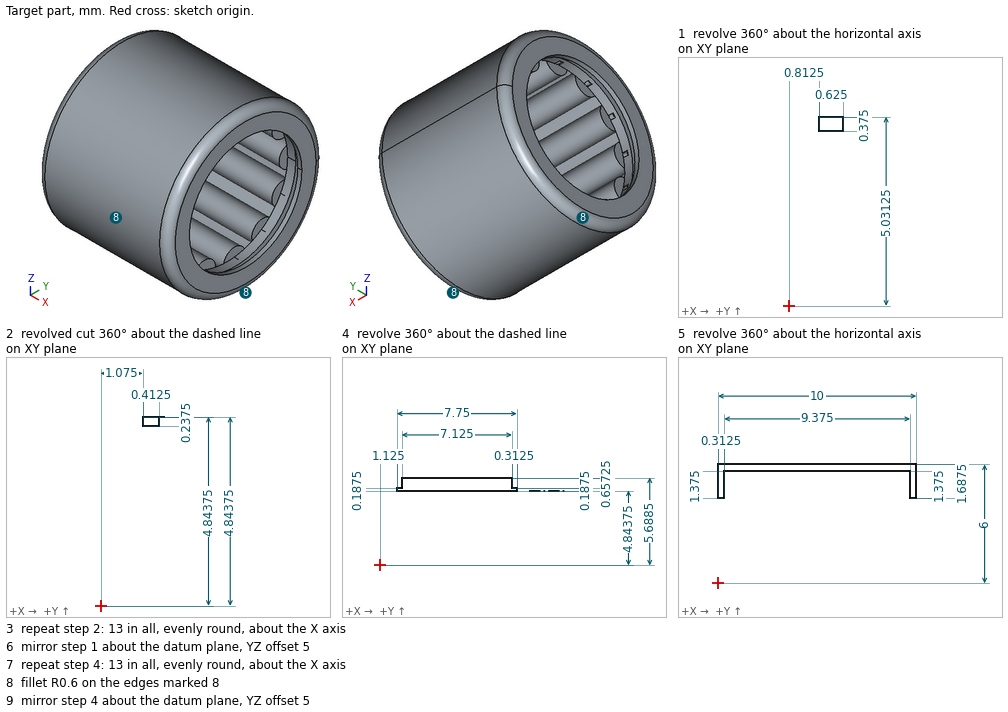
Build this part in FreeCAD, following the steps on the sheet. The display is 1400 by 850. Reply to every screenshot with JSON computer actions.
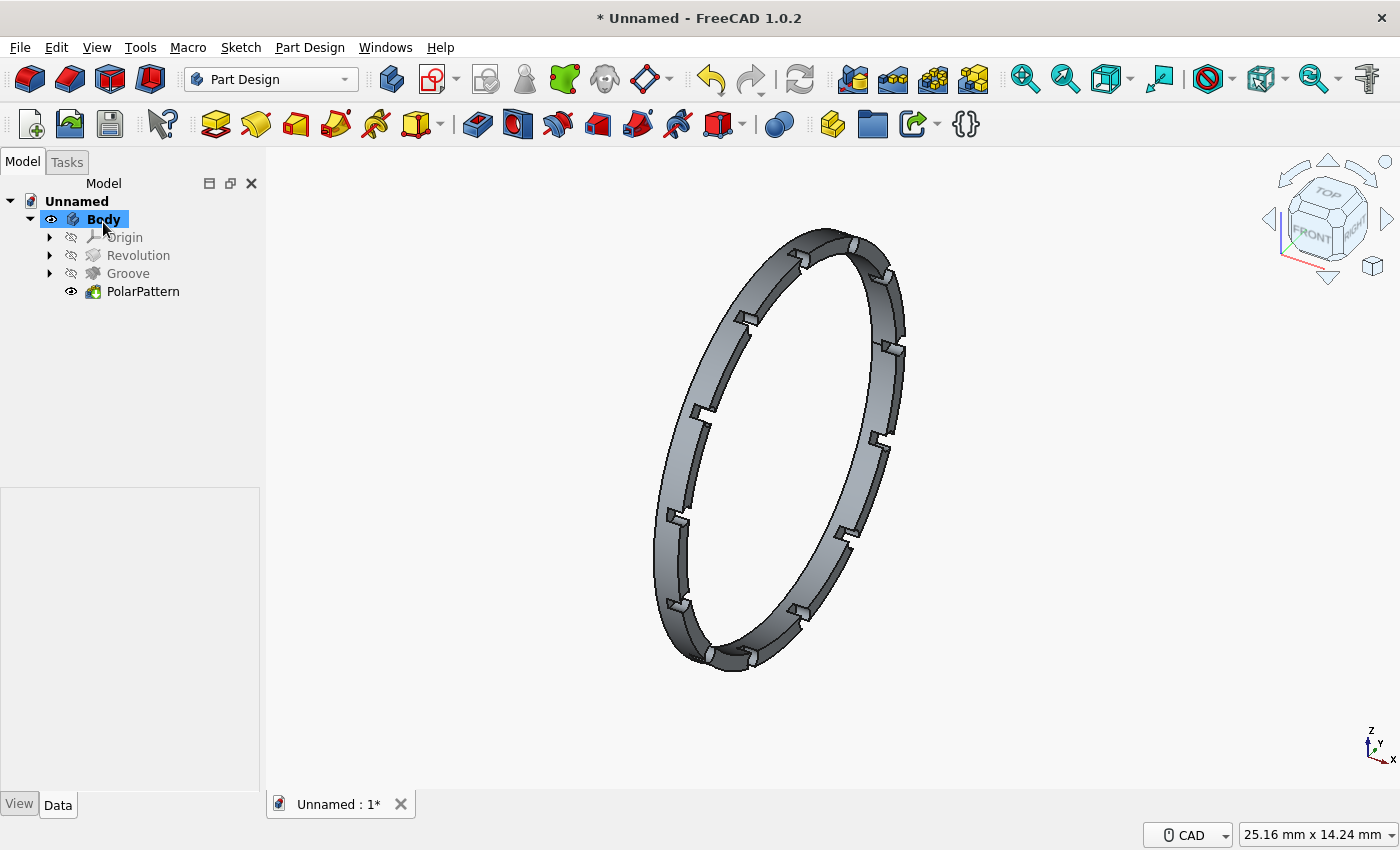
{"action": "left_click", "coordinate": [432, 80]}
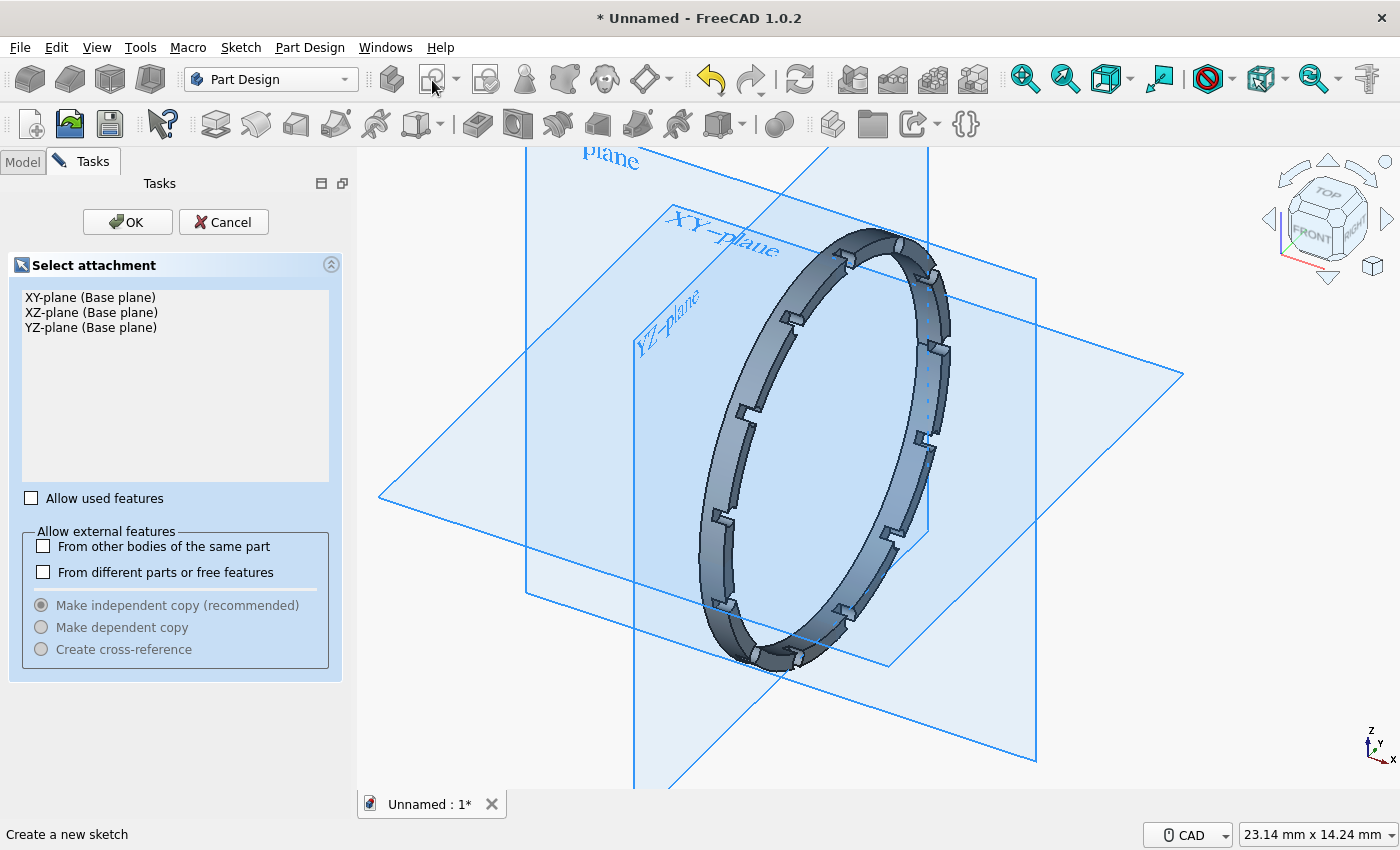
{"action": "left_click", "coordinate": [82, 298]}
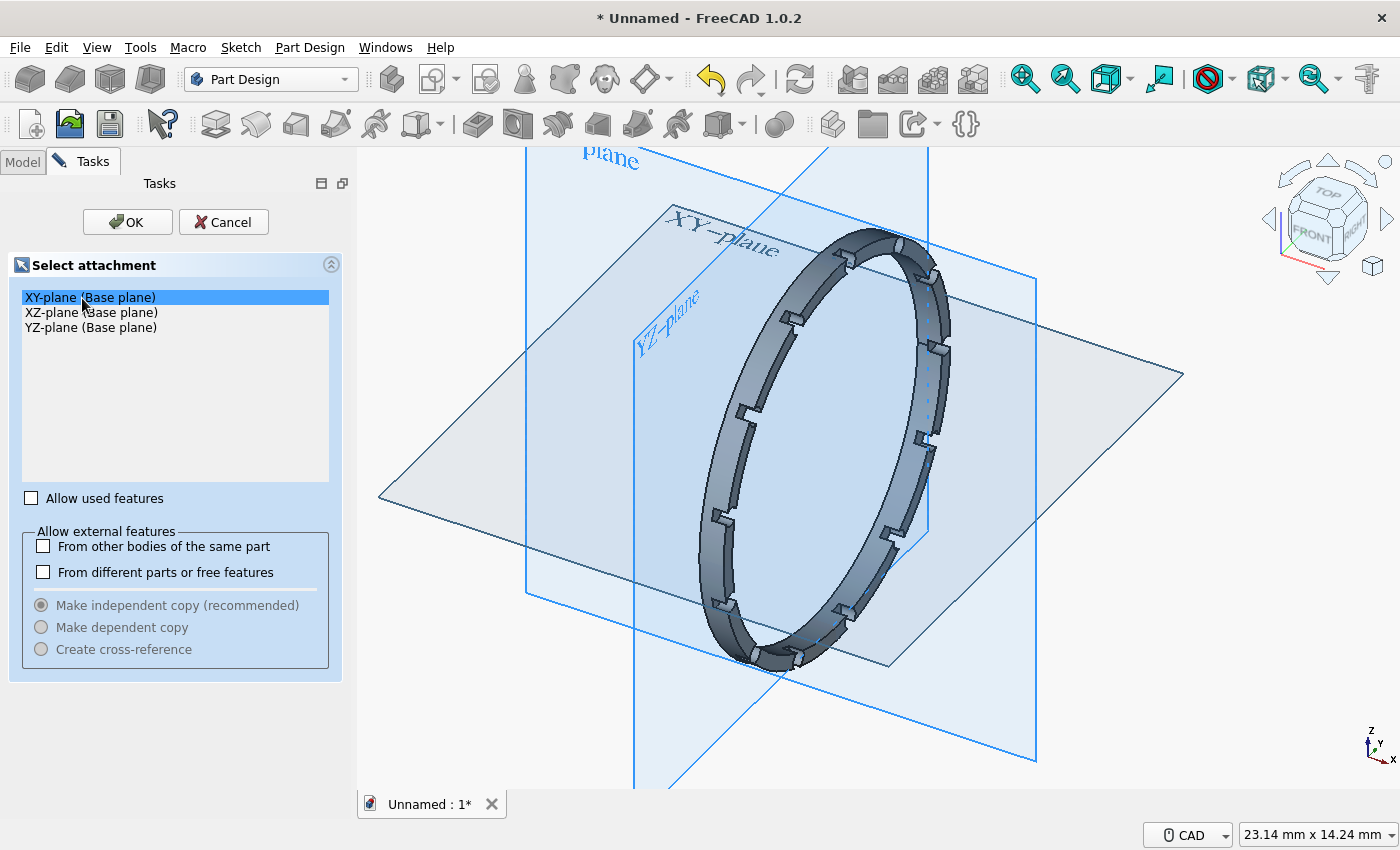
{"action": "left_click", "coordinate": [128, 222]}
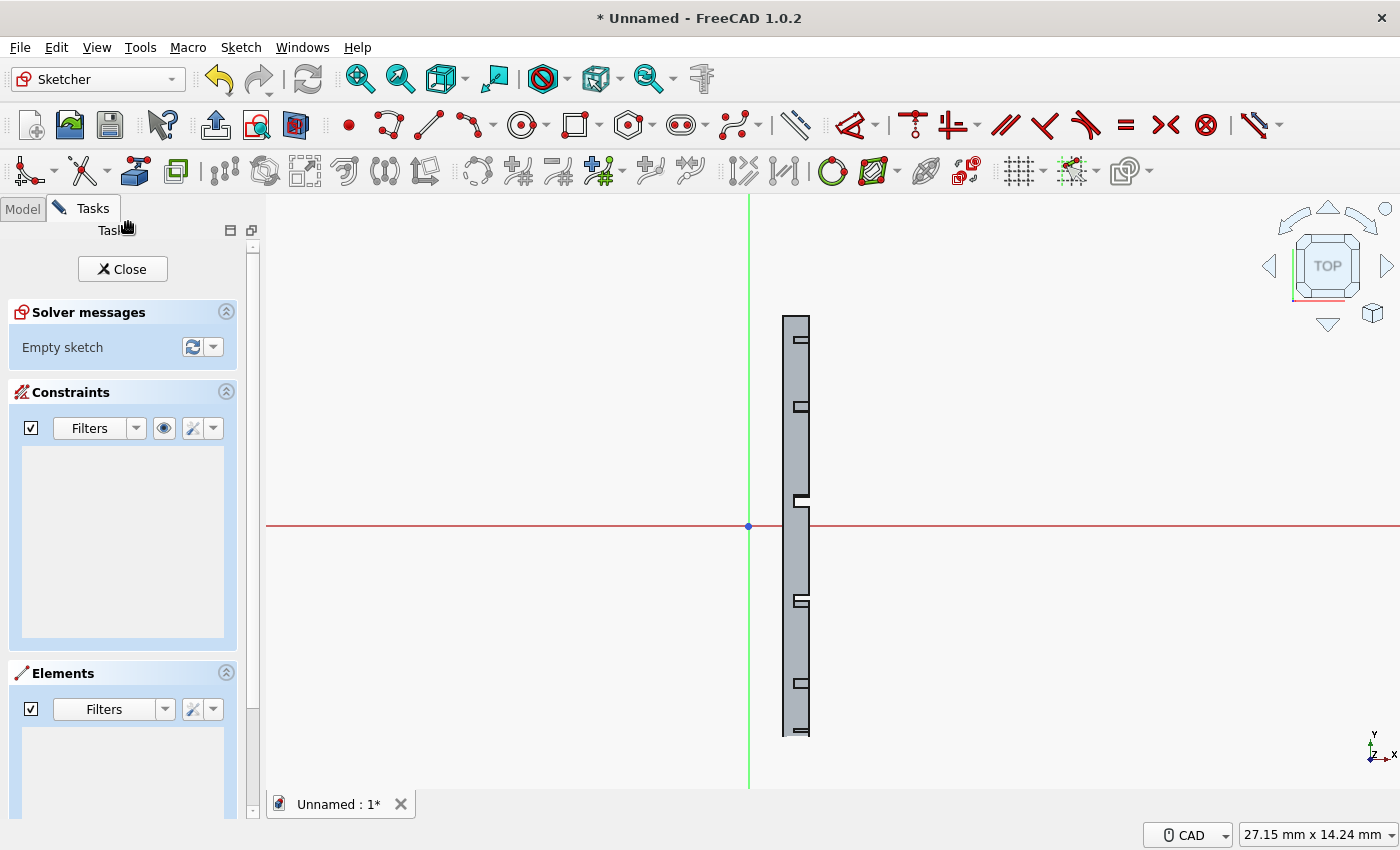
{"action": "key", "text": "q s"}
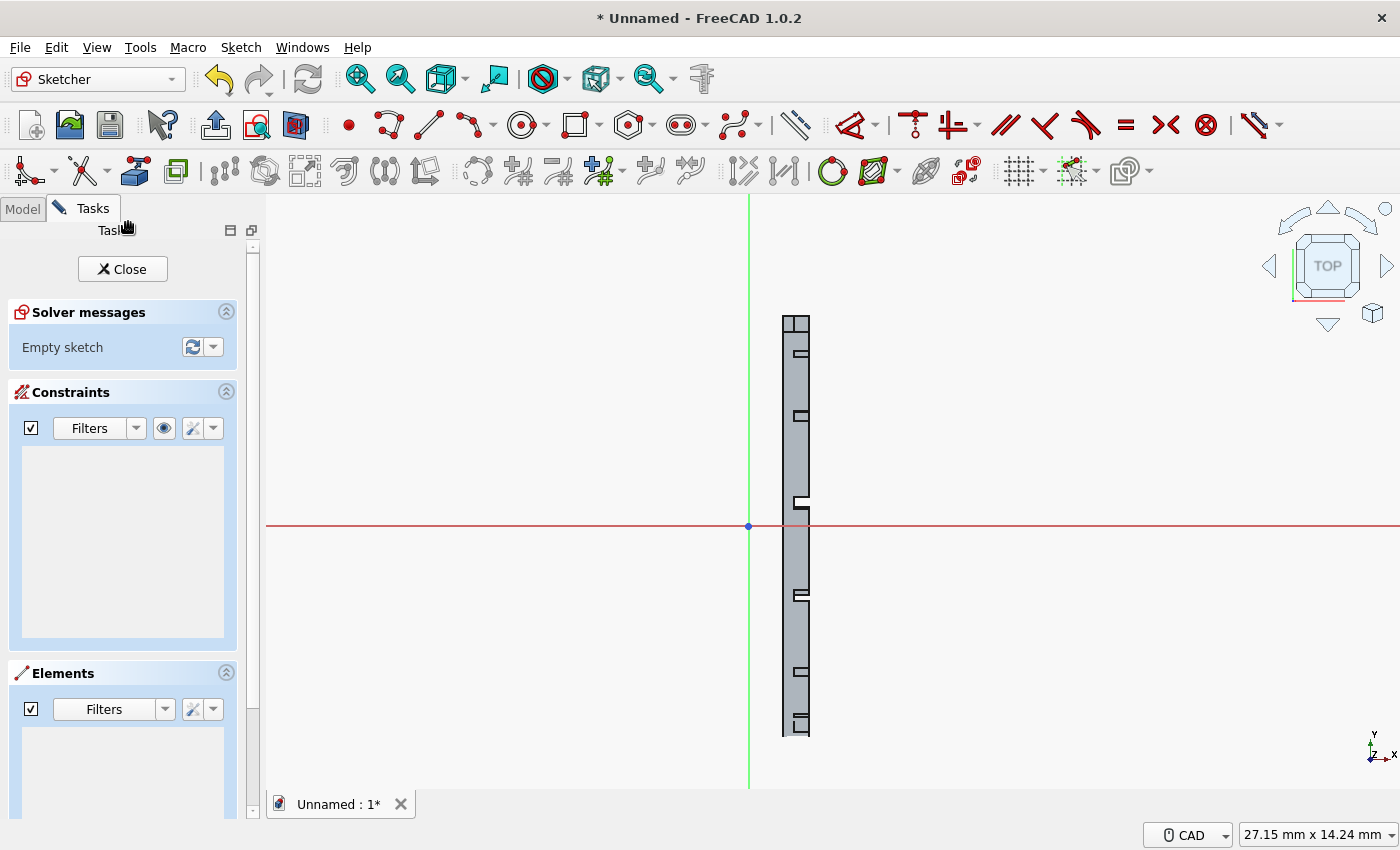
{"action": "scroll", "coordinate": [294, 761], "scroll_direction": "down", "scroll_amount": 1}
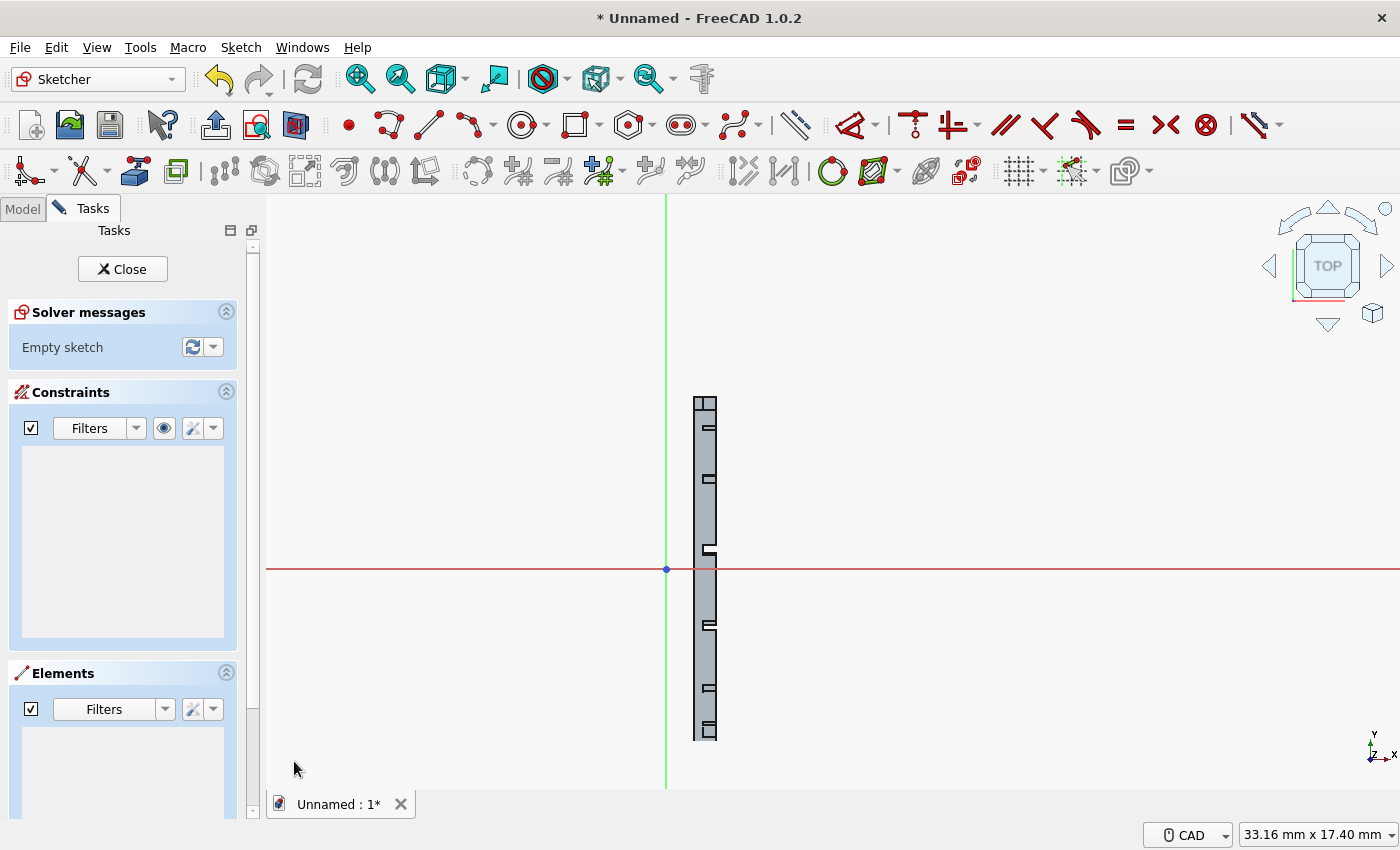
{"action": "scroll", "coordinate": [1088, 432], "scroll_direction": "up", "scroll_amount": 2}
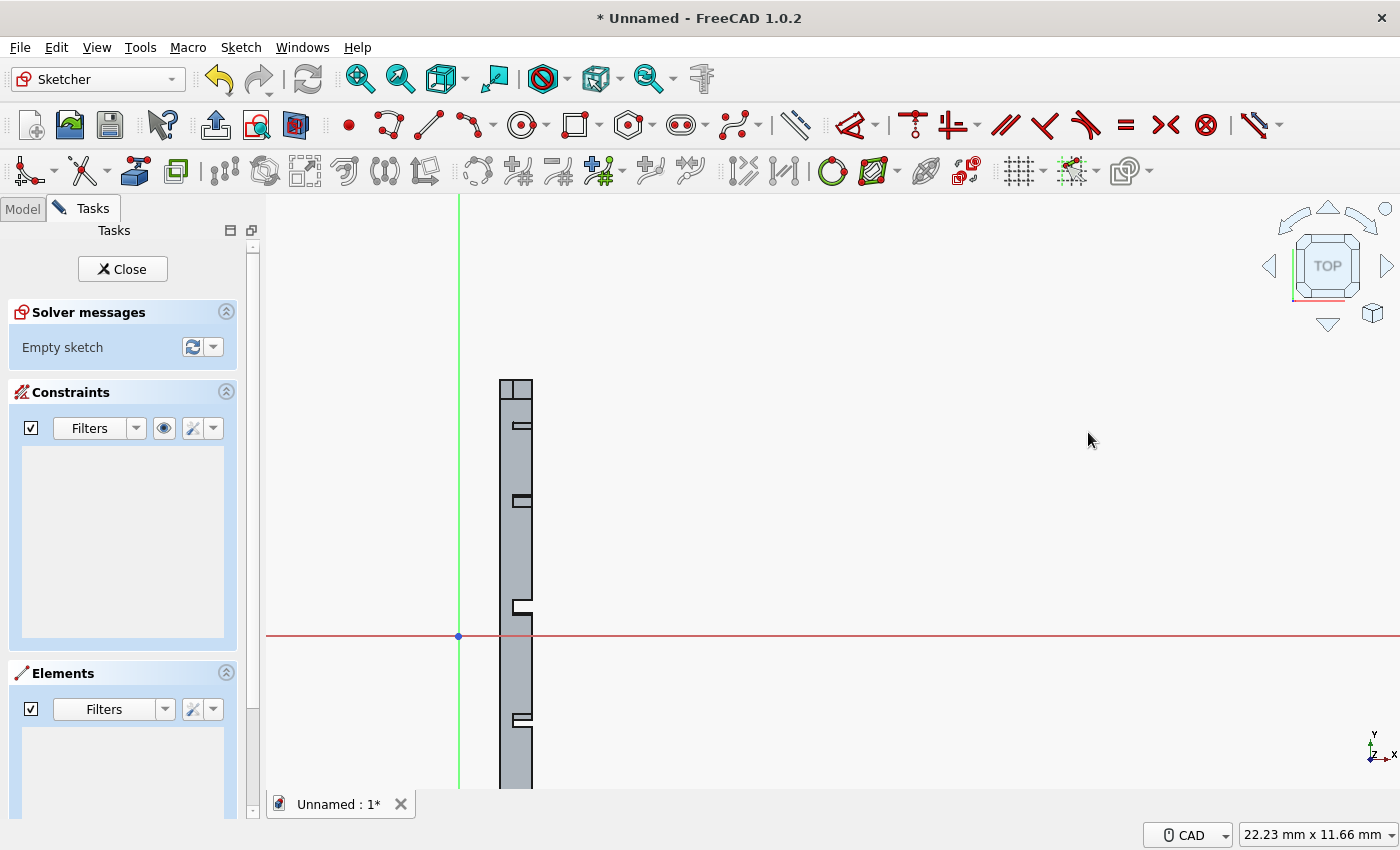
{"action": "key", "text": "g m"}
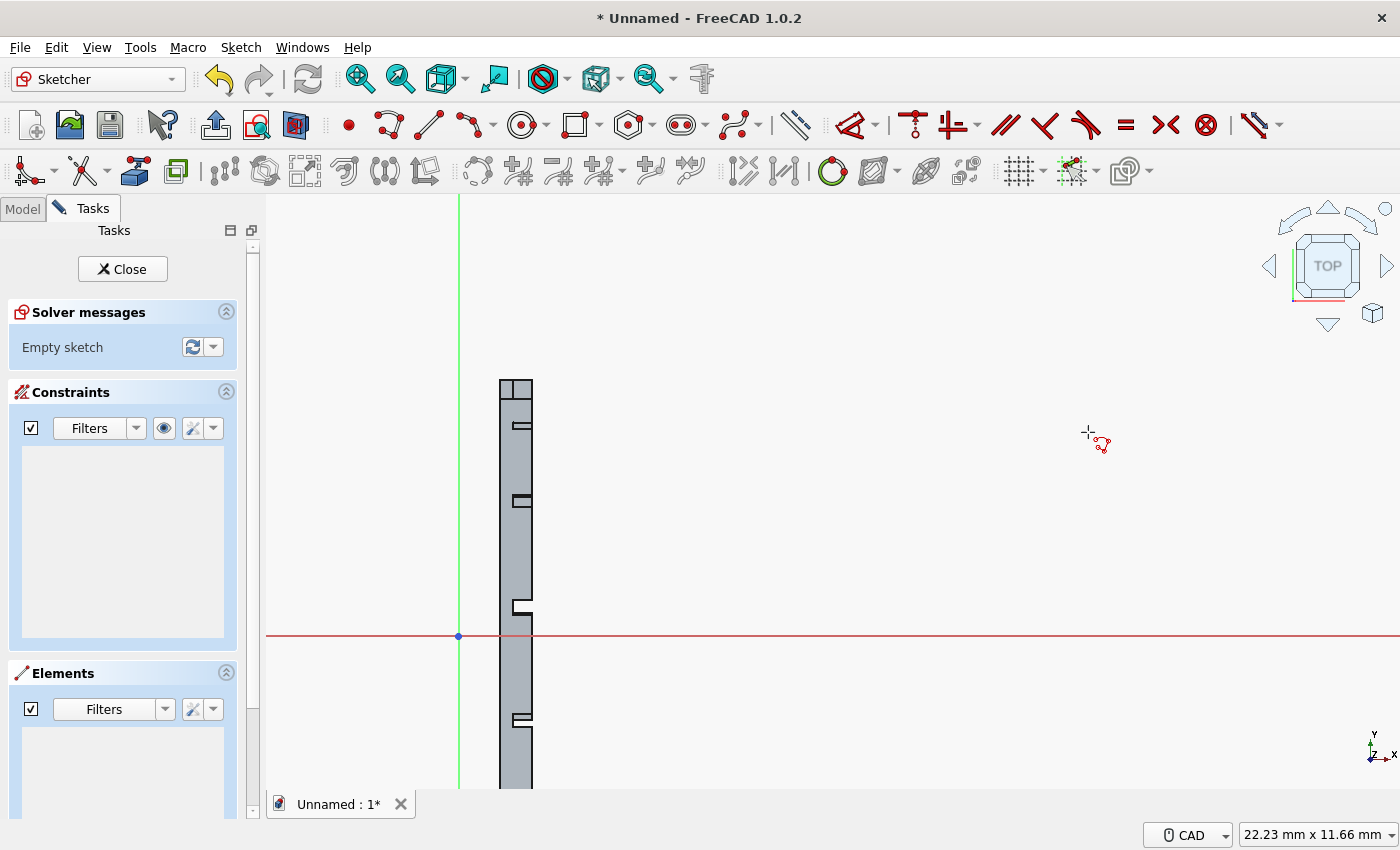
{"action": "left_click", "coordinate": [516, 389]}
{"action": "left_click", "coordinate": [911, 389]}